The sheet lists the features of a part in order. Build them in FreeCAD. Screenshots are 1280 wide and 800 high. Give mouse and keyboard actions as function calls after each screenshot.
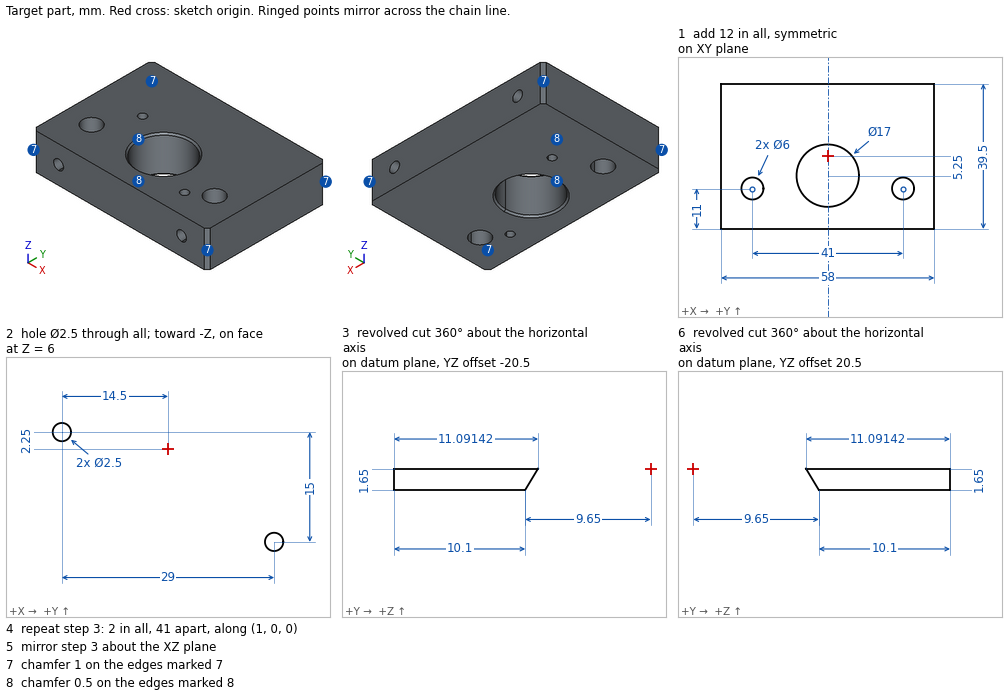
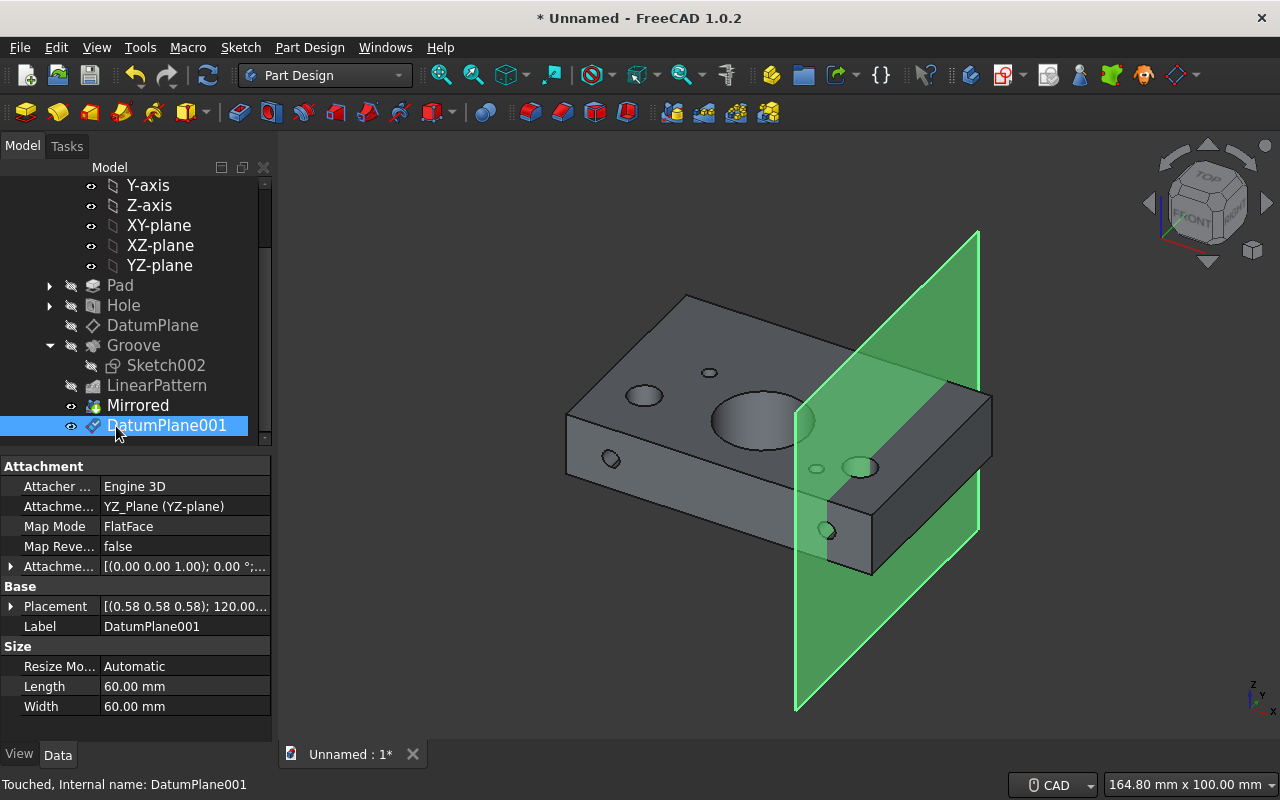
click(1004, 76)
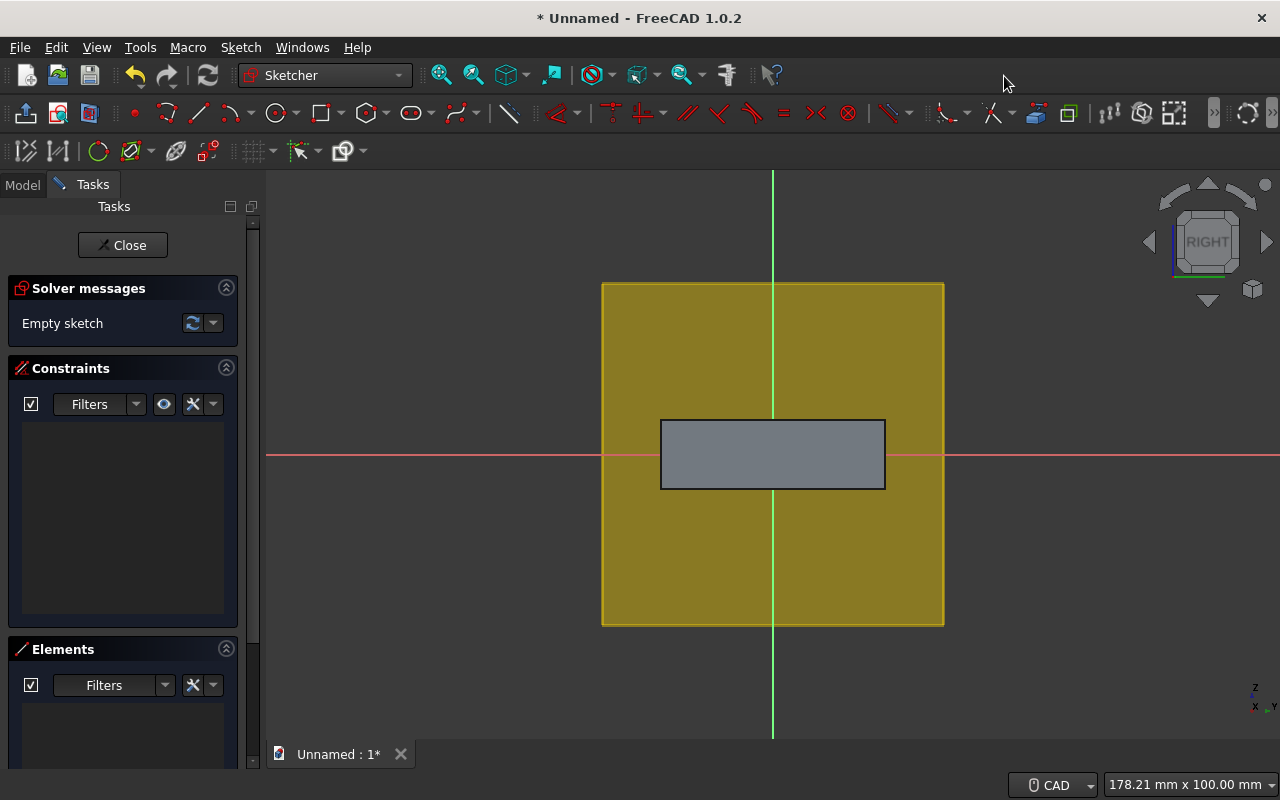
click(90, 114)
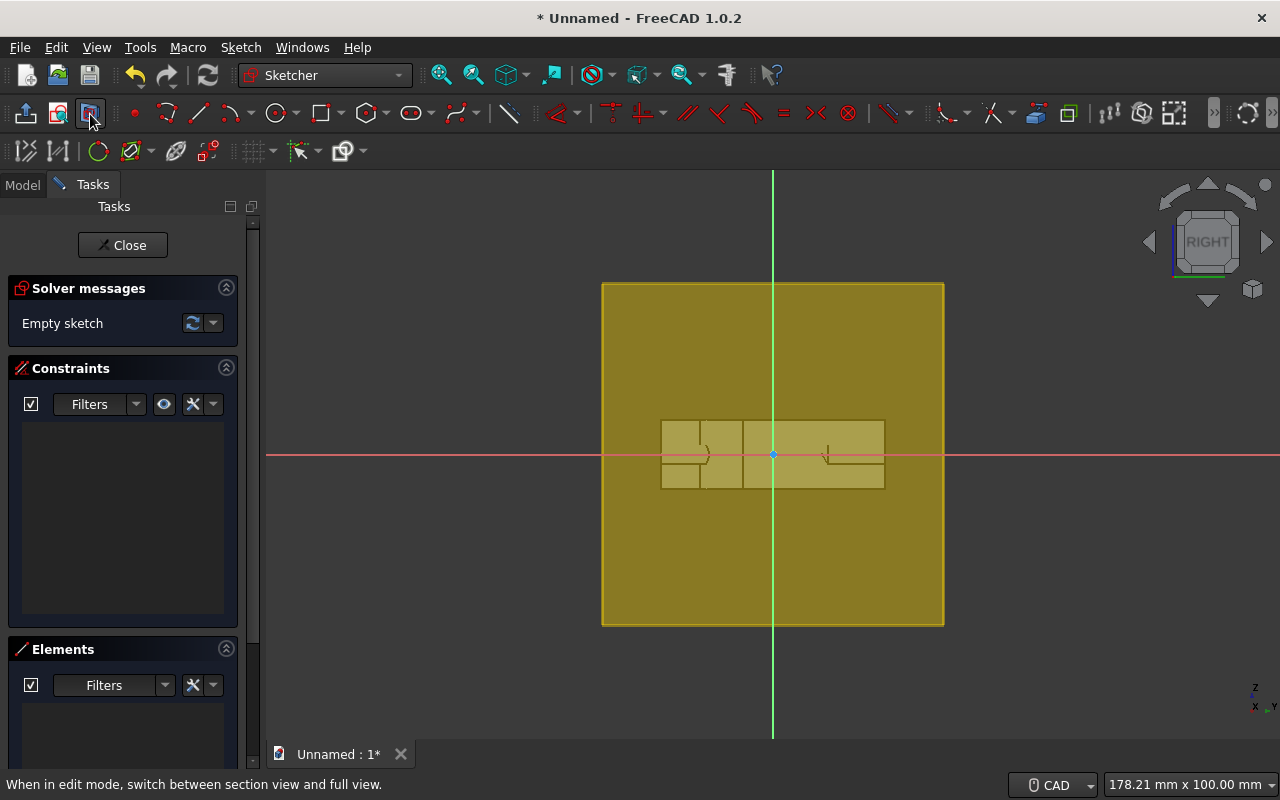
scroll(861, 460, up, 8)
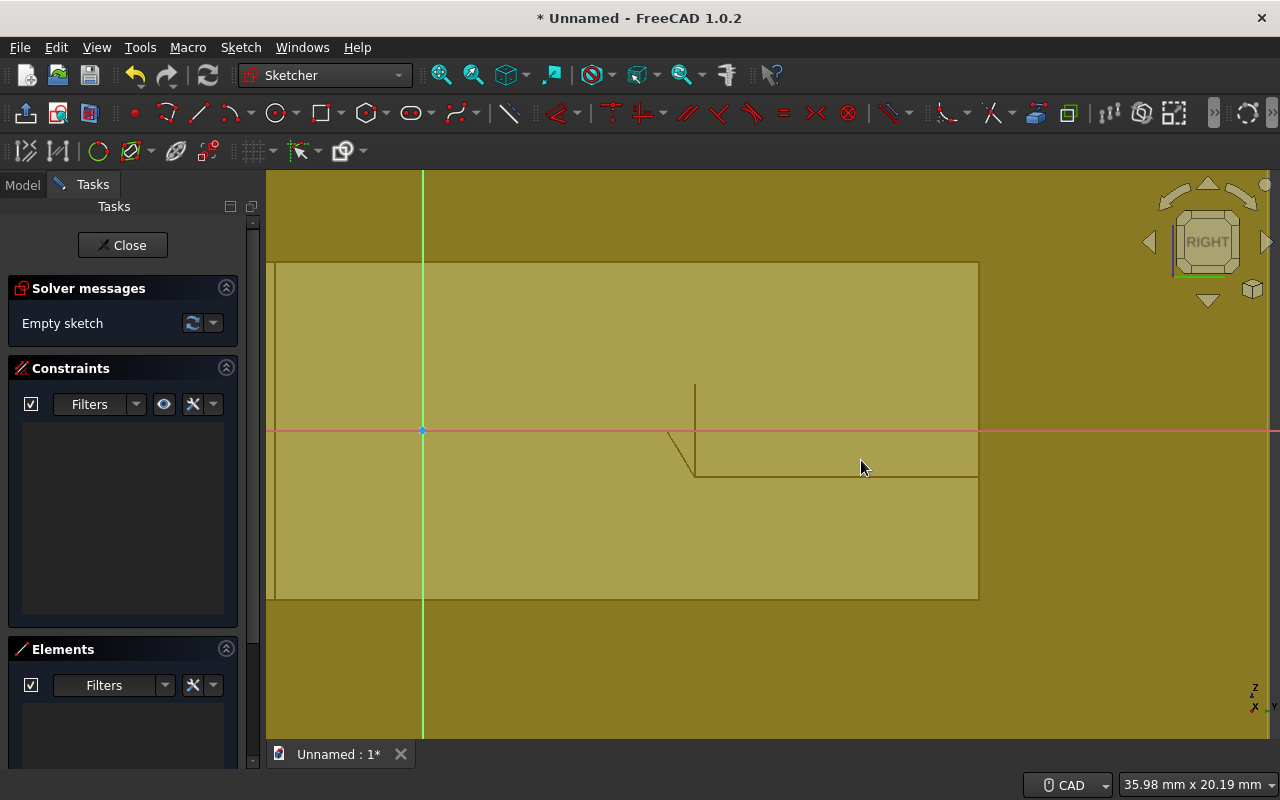
click(168, 114)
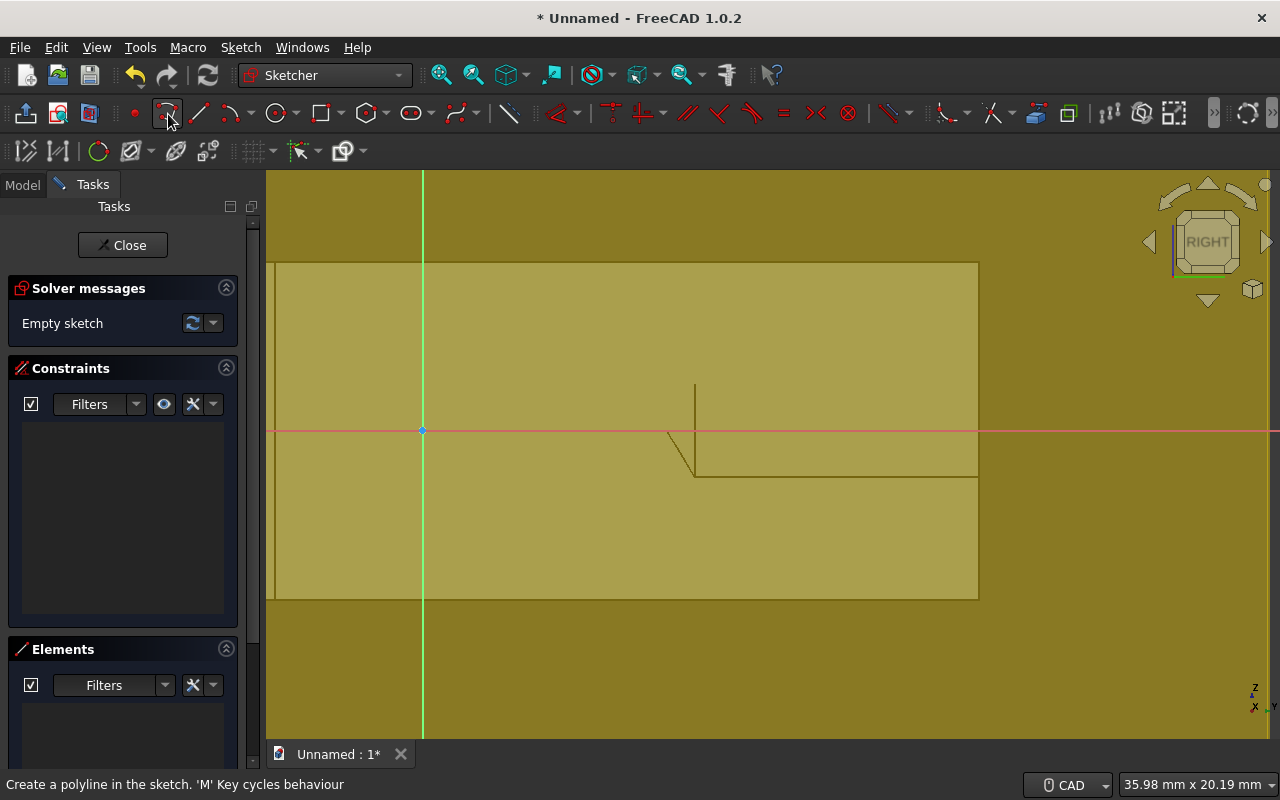
click(667, 431)
click(695, 477)
click(979, 477)
click(979, 440)
click(667, 431)
key(Escape)
key(Escape)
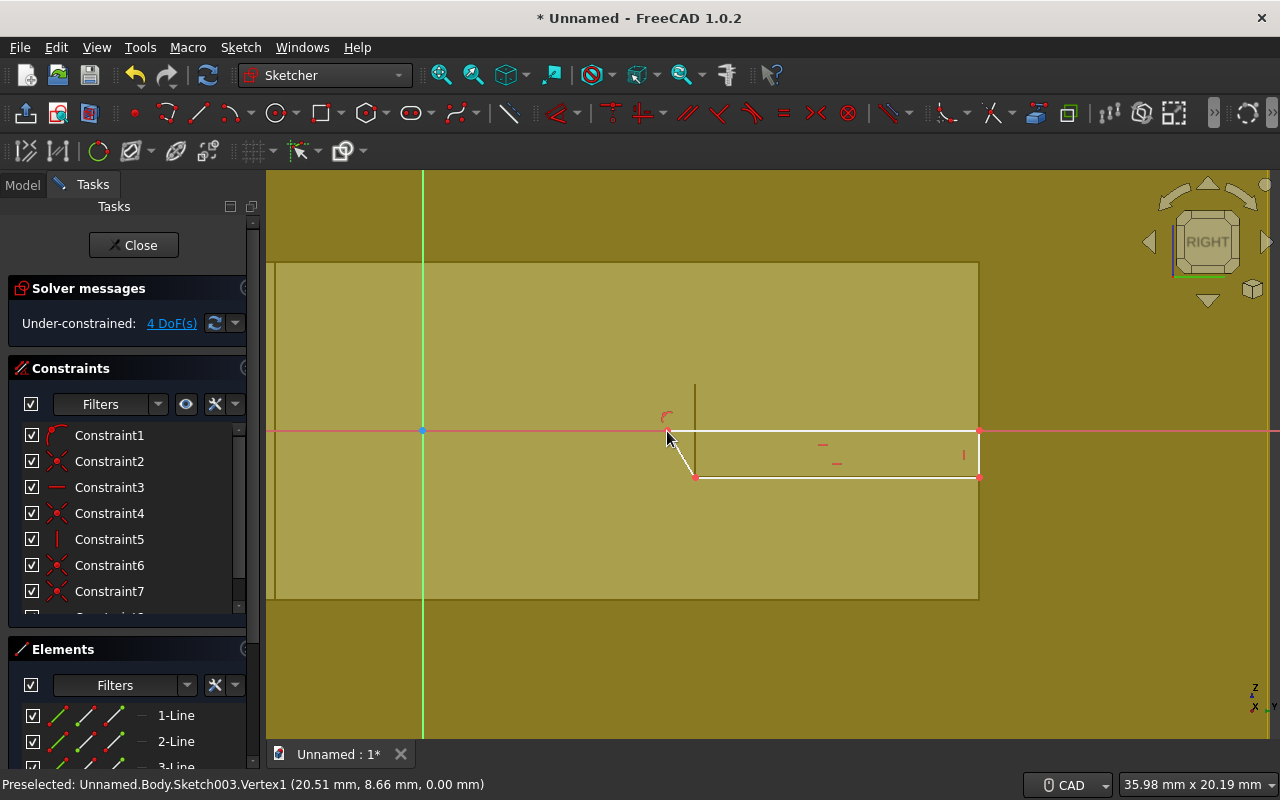
key(d)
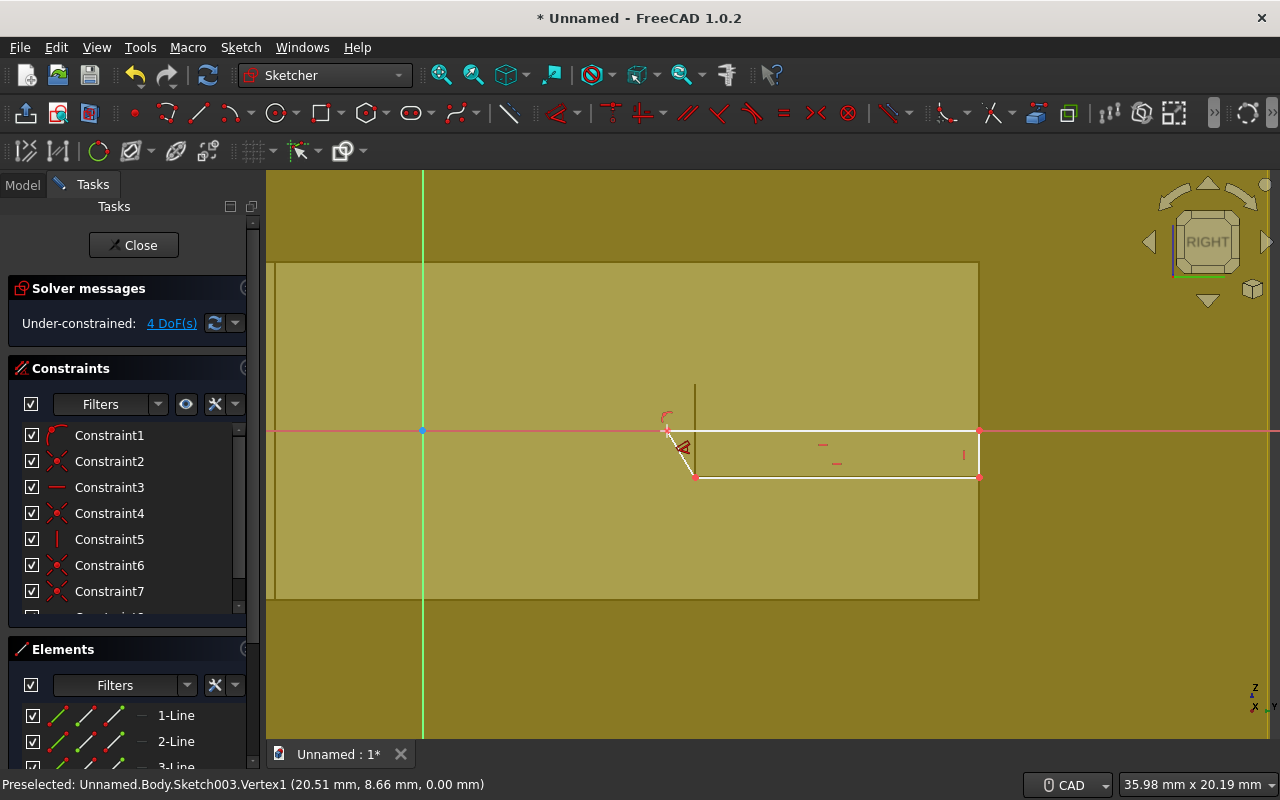
click(780, 478)
click(837, 512)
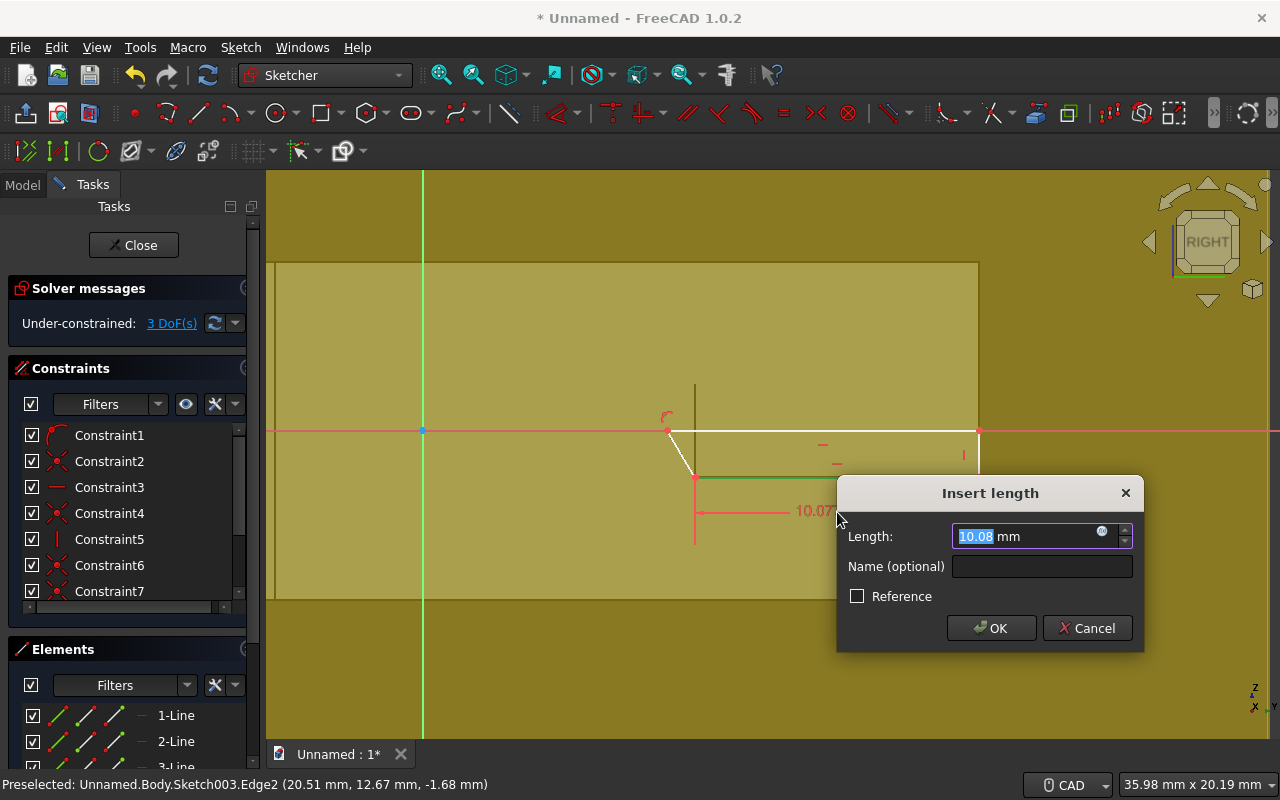
text(10.1)
key(Return)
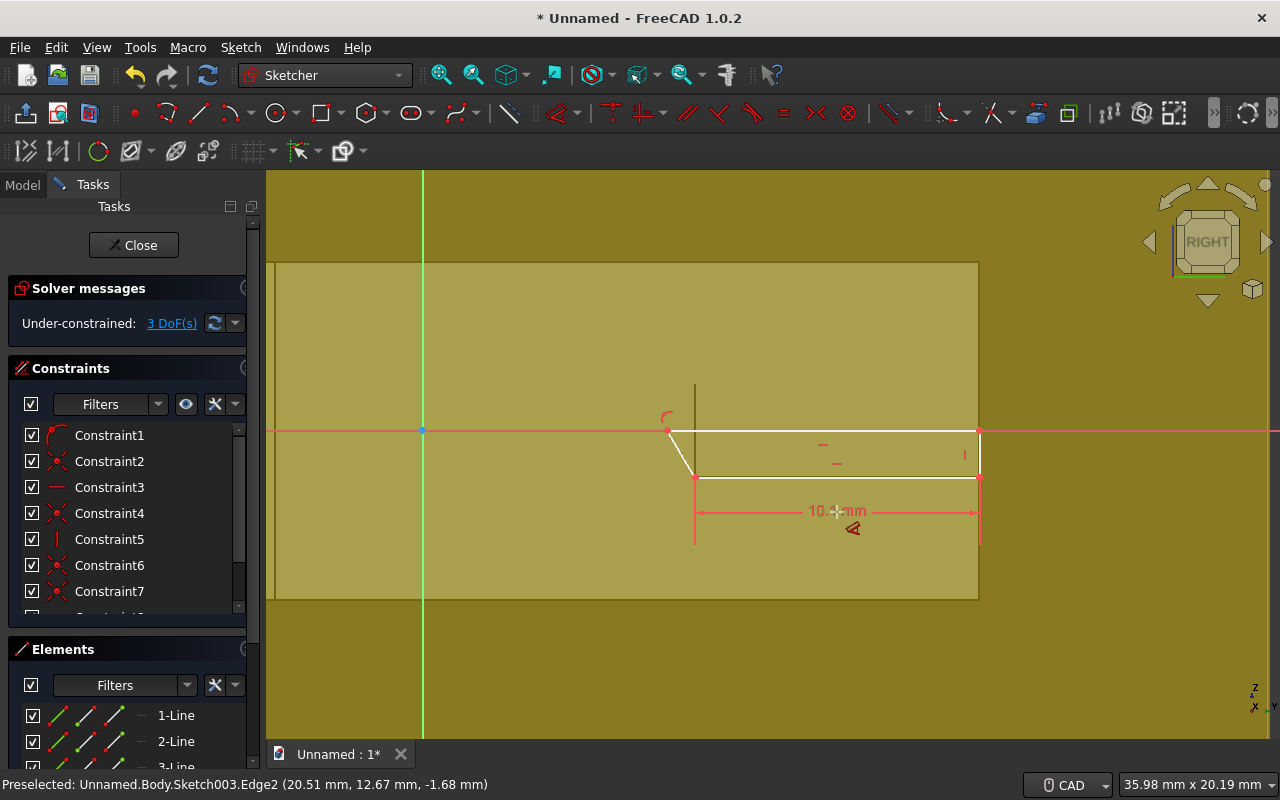
click(980, 464)
click(1014, 454)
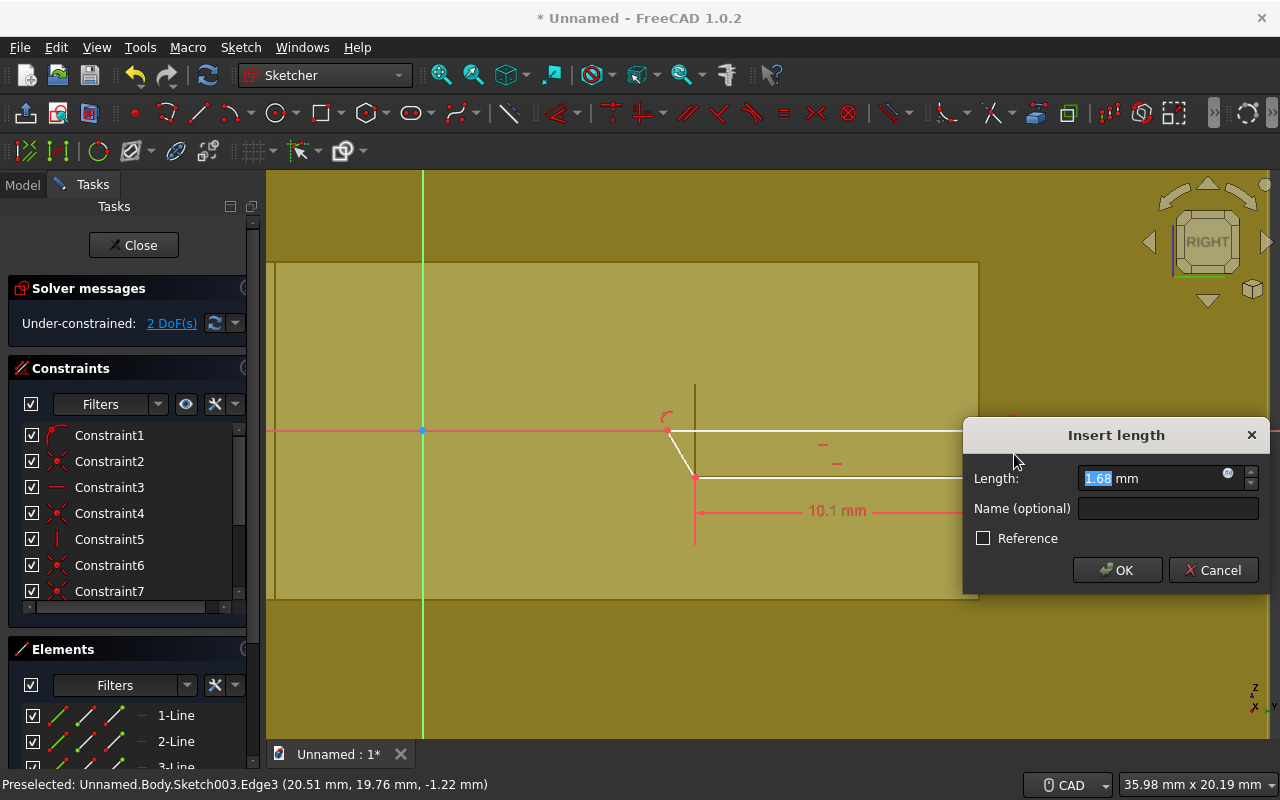
text(1.65)
key(Return)